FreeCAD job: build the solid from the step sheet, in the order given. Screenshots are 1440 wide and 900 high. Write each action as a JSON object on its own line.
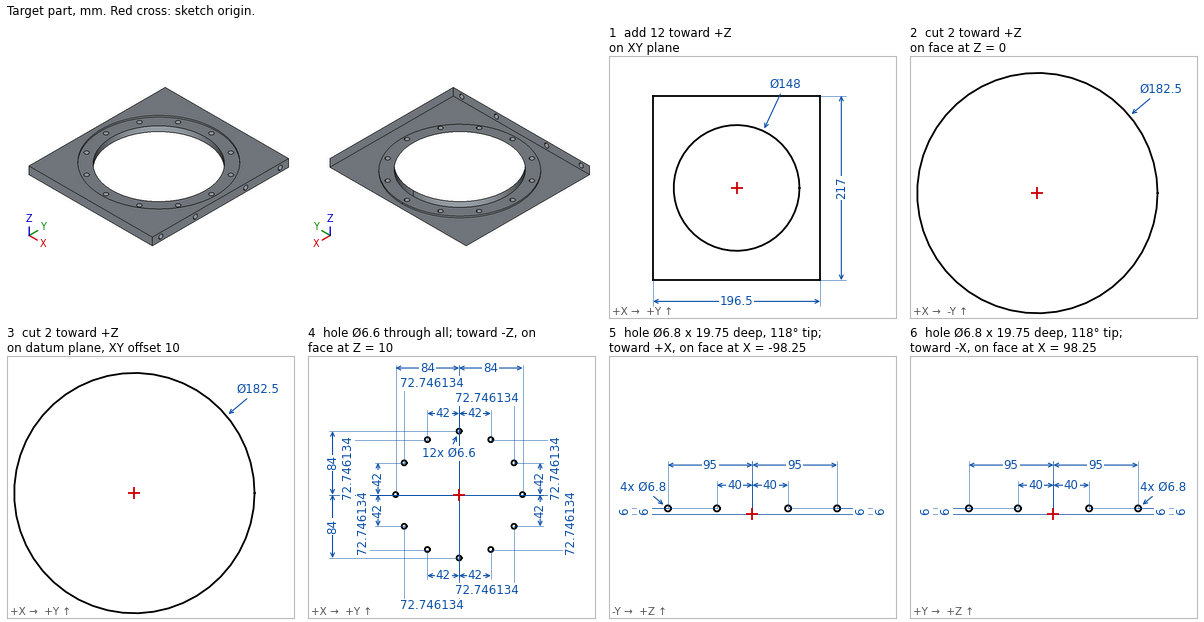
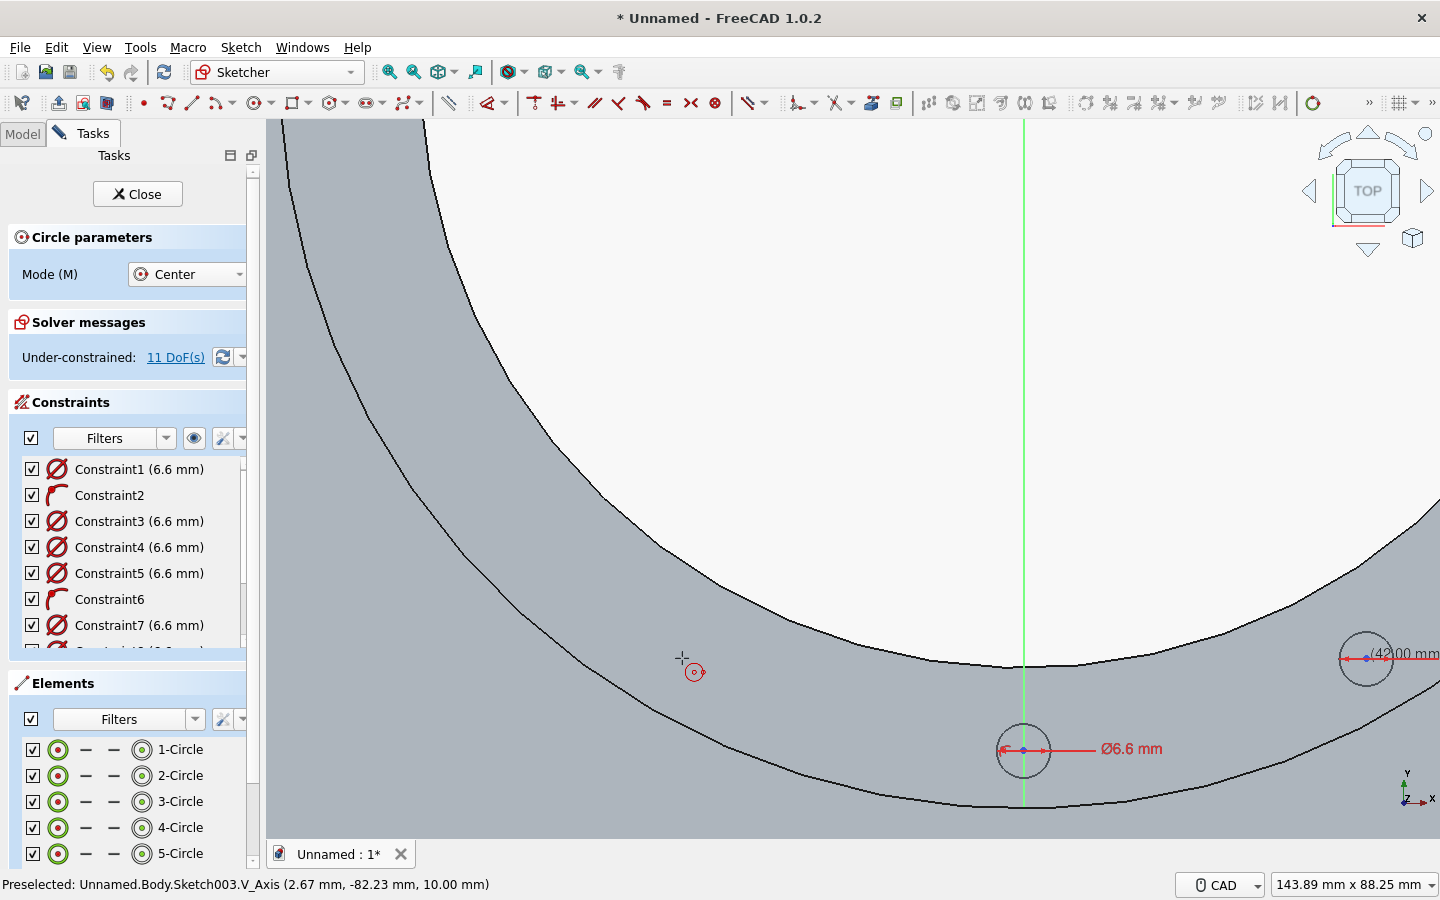
{"action": "left_click", "coordinate": [681, 658]}
{"action": "mouse_move", "coordinate": [700, 639]}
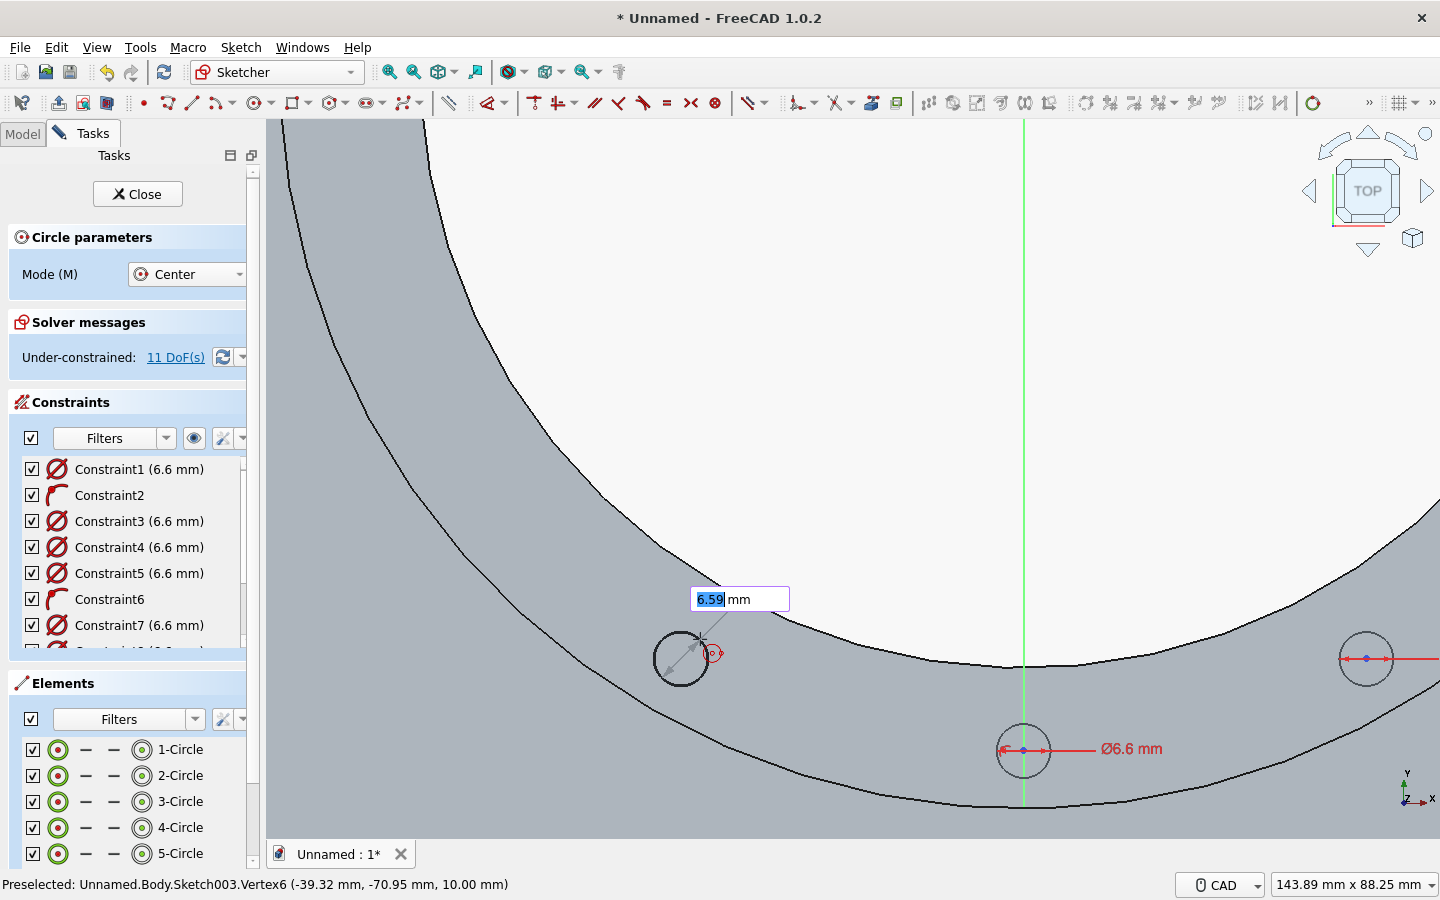
{"action": "type", "text": "6.6"}
{"action": "key", "text": "Return"}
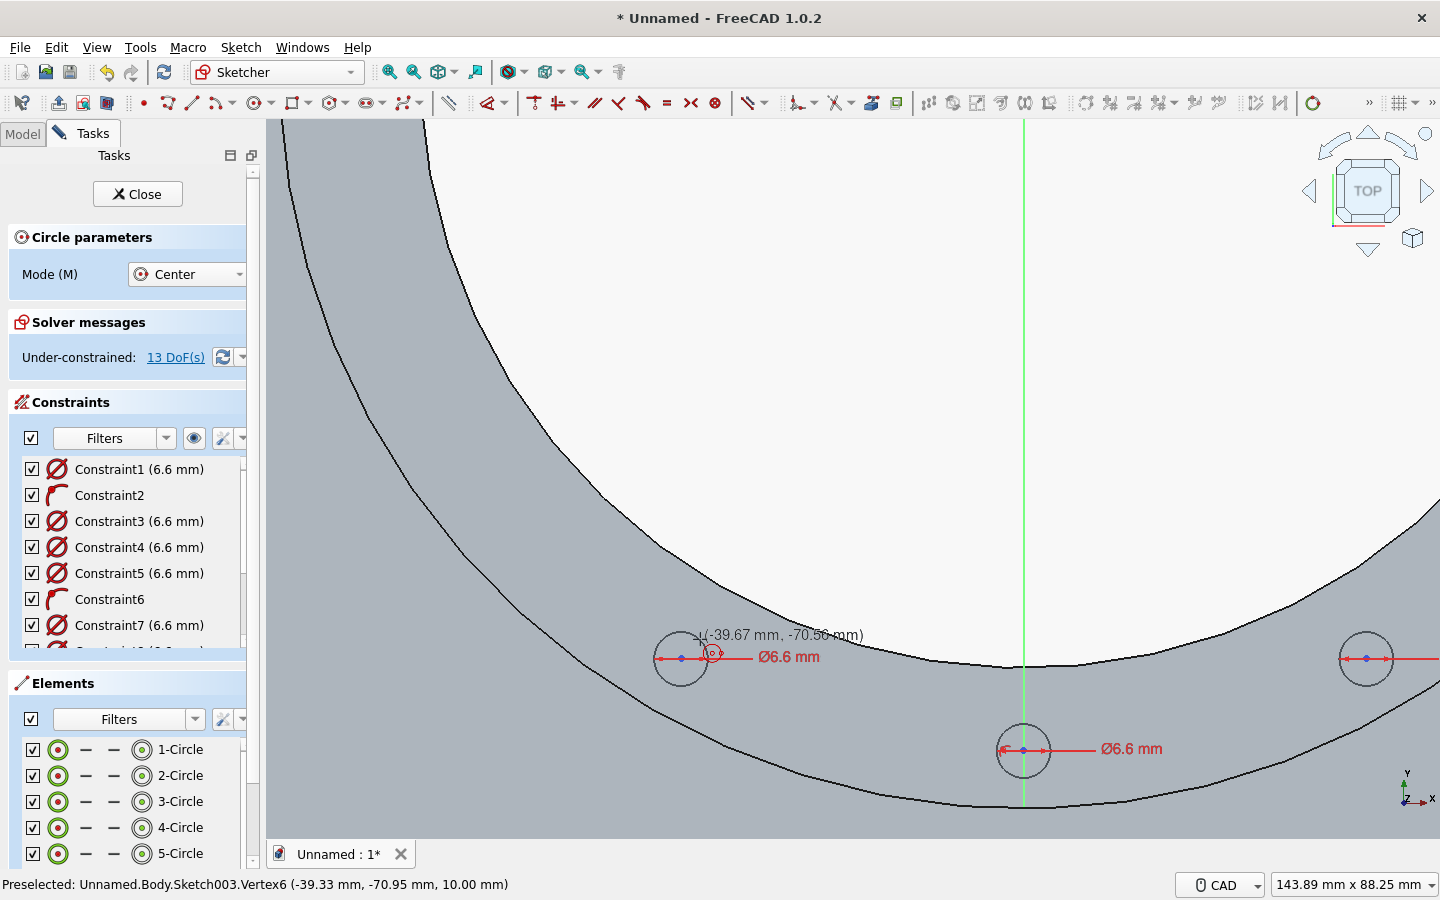
{"action": "left_click", "coordinate": [430, 407]}
{"action": "mouse_move", "coordinate": [449, 388]}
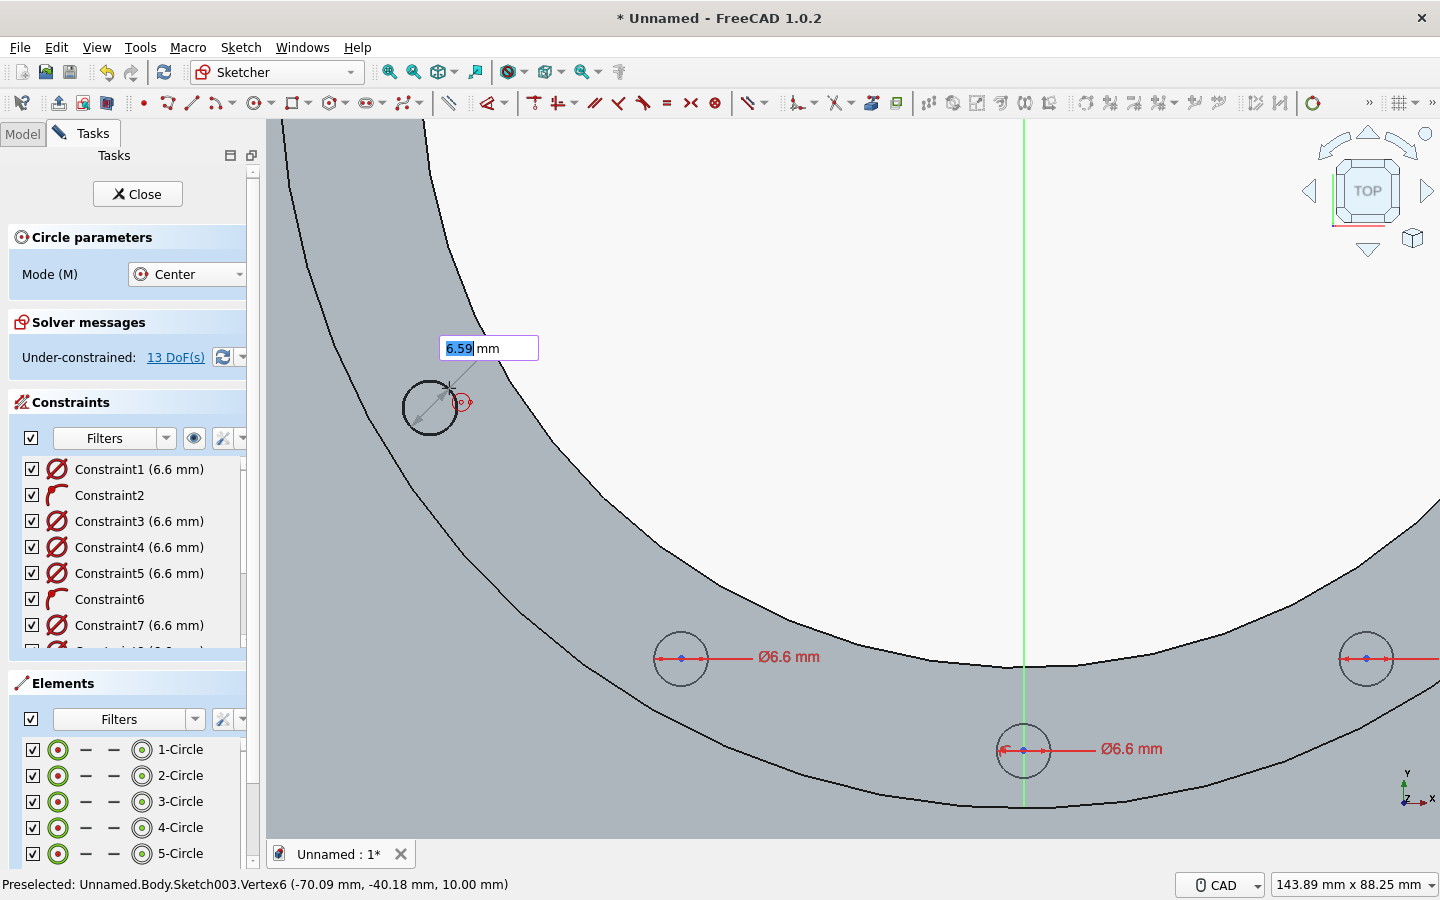
{"action": "type", "text": "6.6"}
{"action": "key", "text": "Return"}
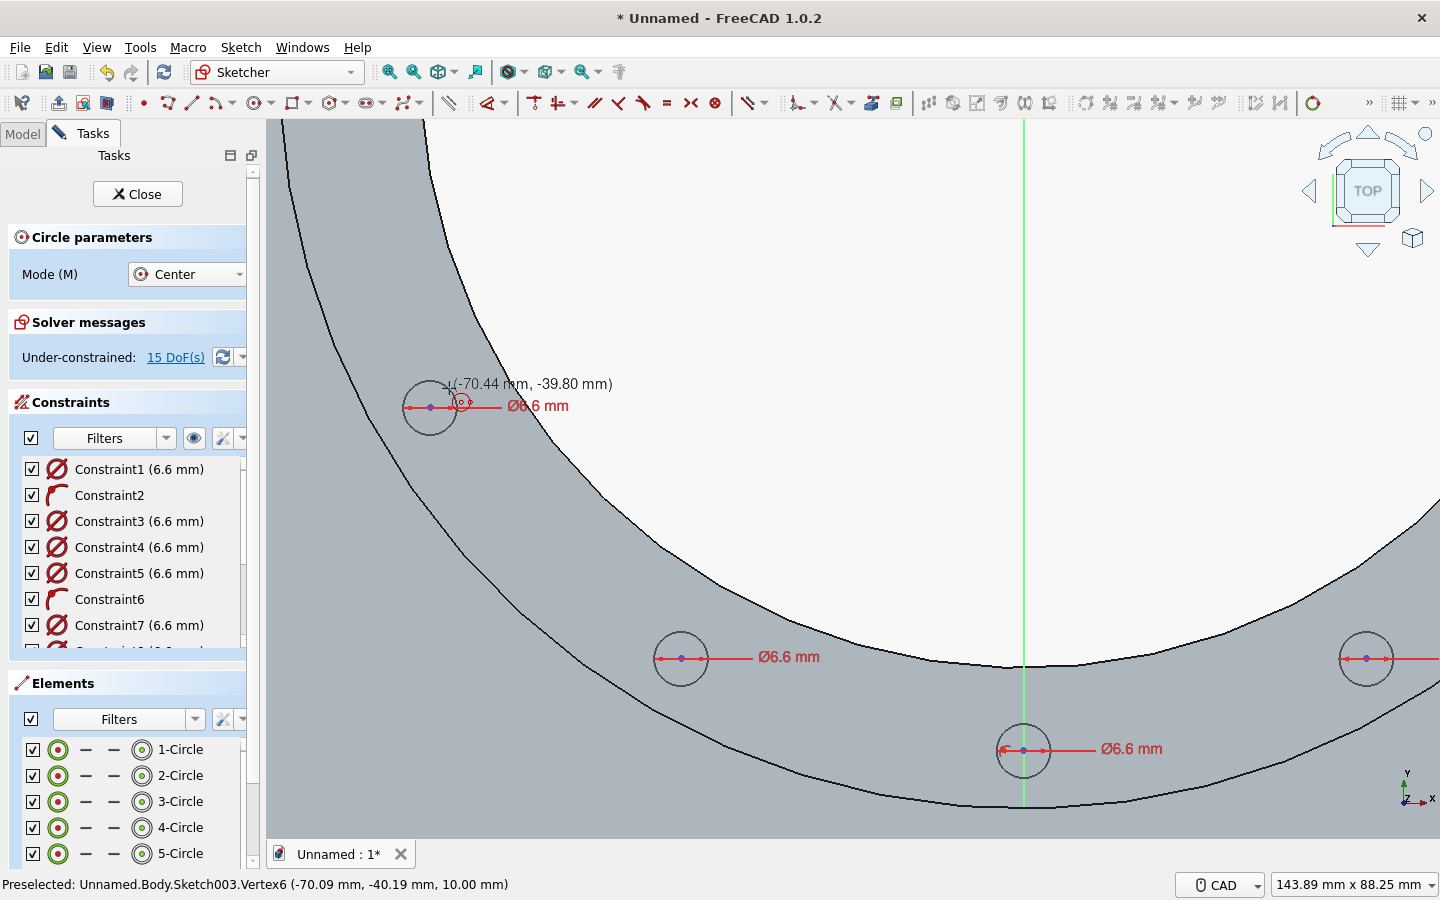
{"action": "scroll", "coordinate": [681, 658], "scroll_direction": "down", "scroll_amount": 6}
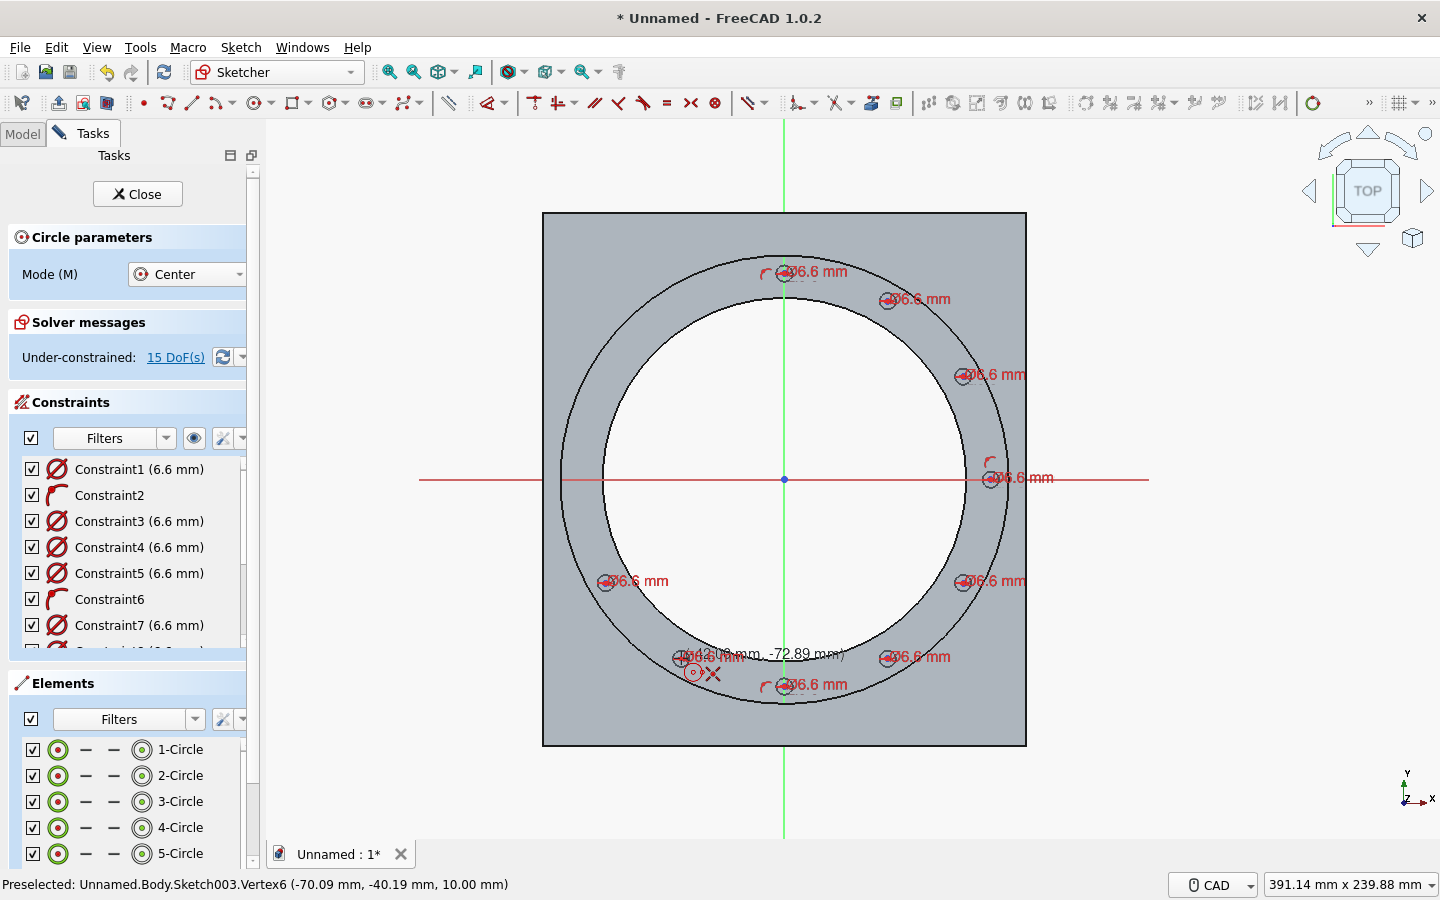
{"action": "scroll", "coordinate": [578, 480], "scroll_direction": "up", "scroll_amount": 6}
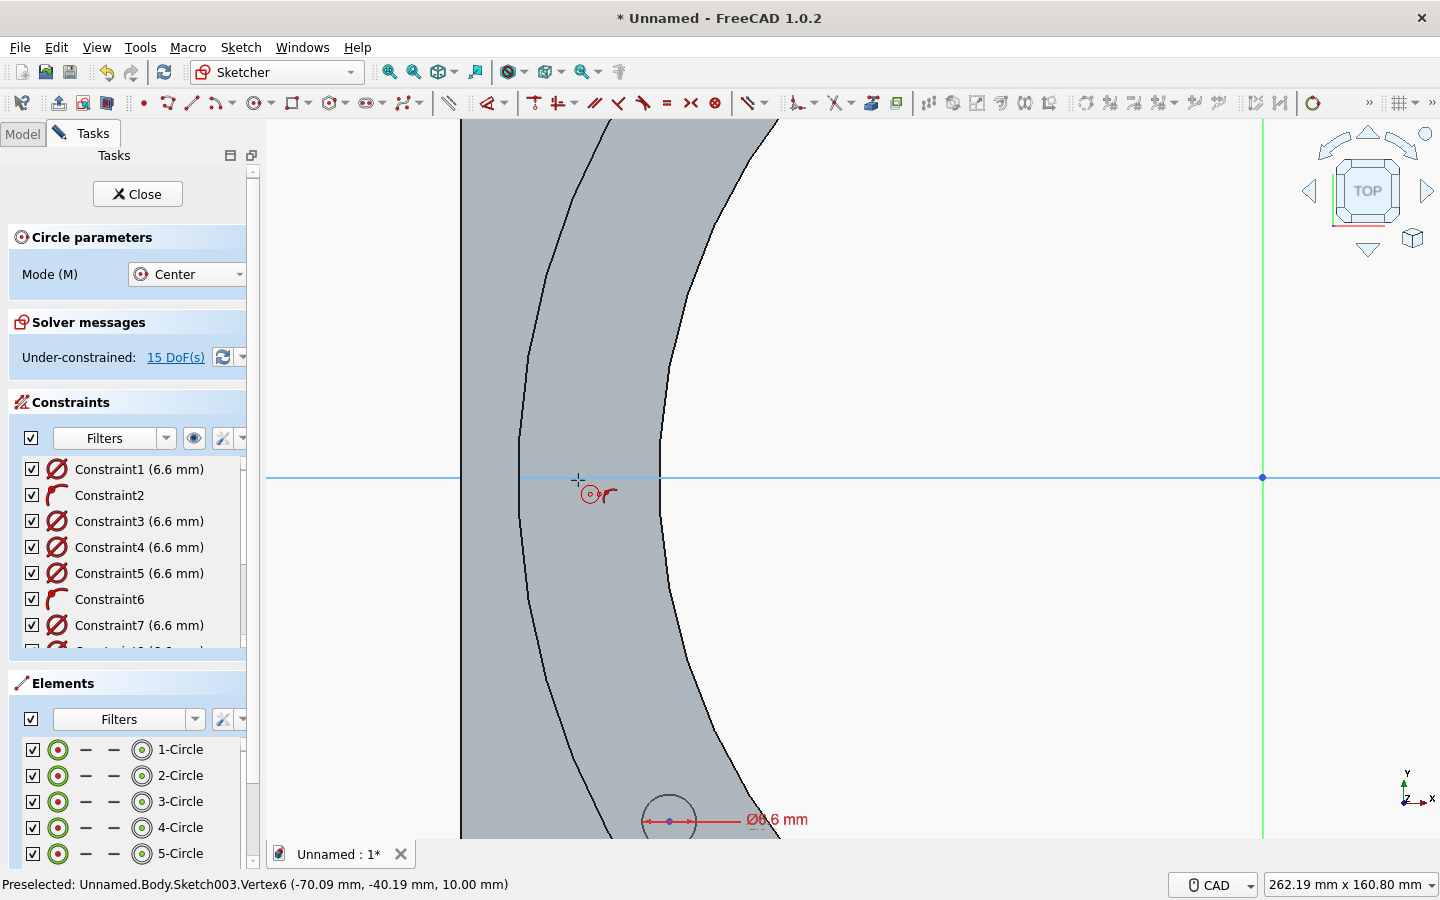
{"action": "left_click", "coordinate": [578, 478]}
{"action": "mouse_move", "coordinate": [597, 459]}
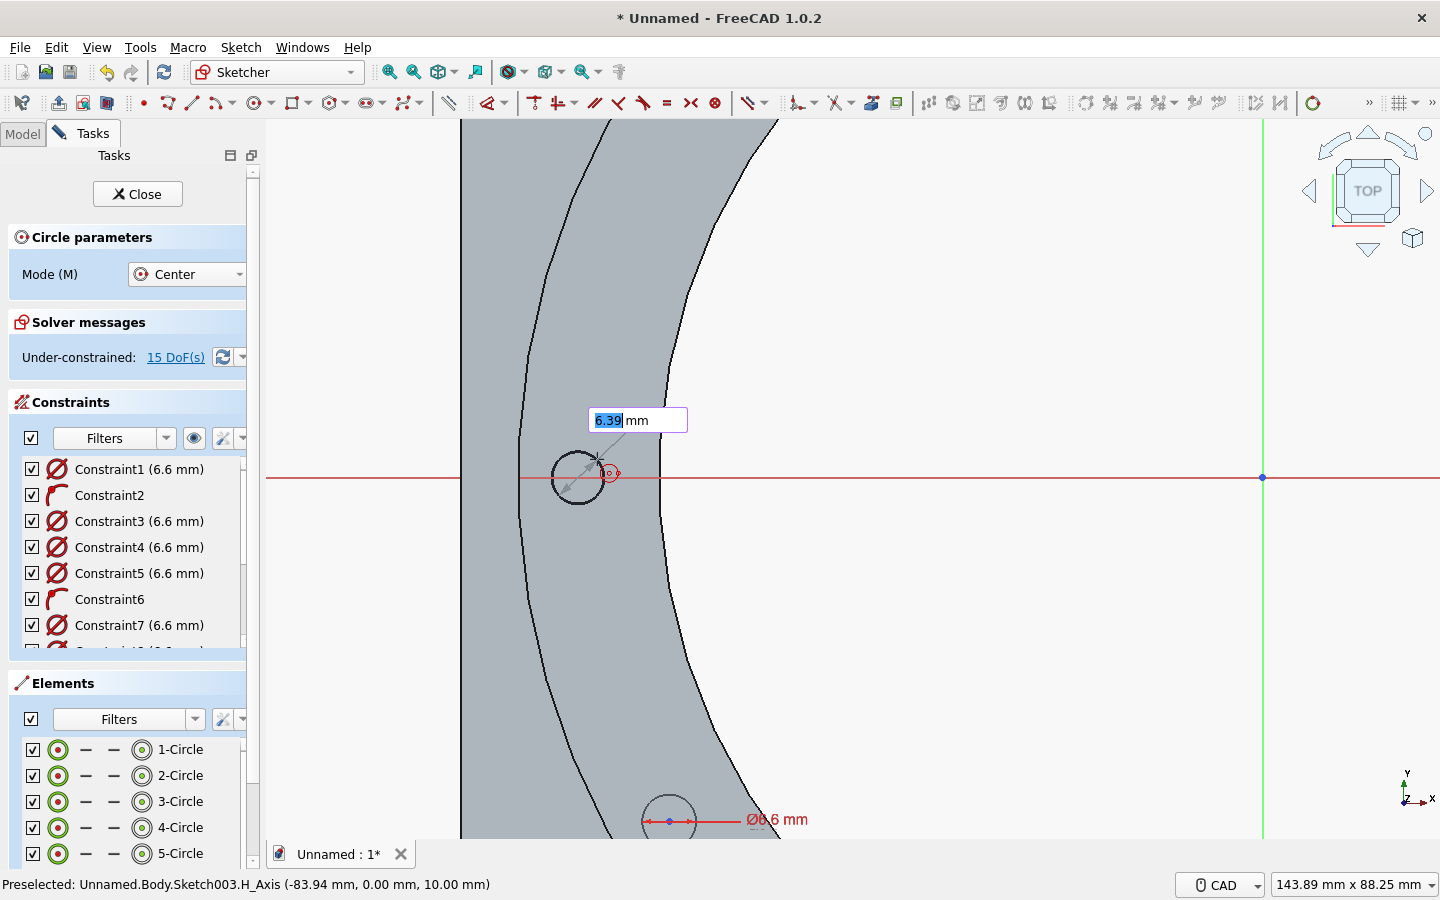
{"action": "type", "text": "6.6"}
{"action": "key", "text": "Return"}